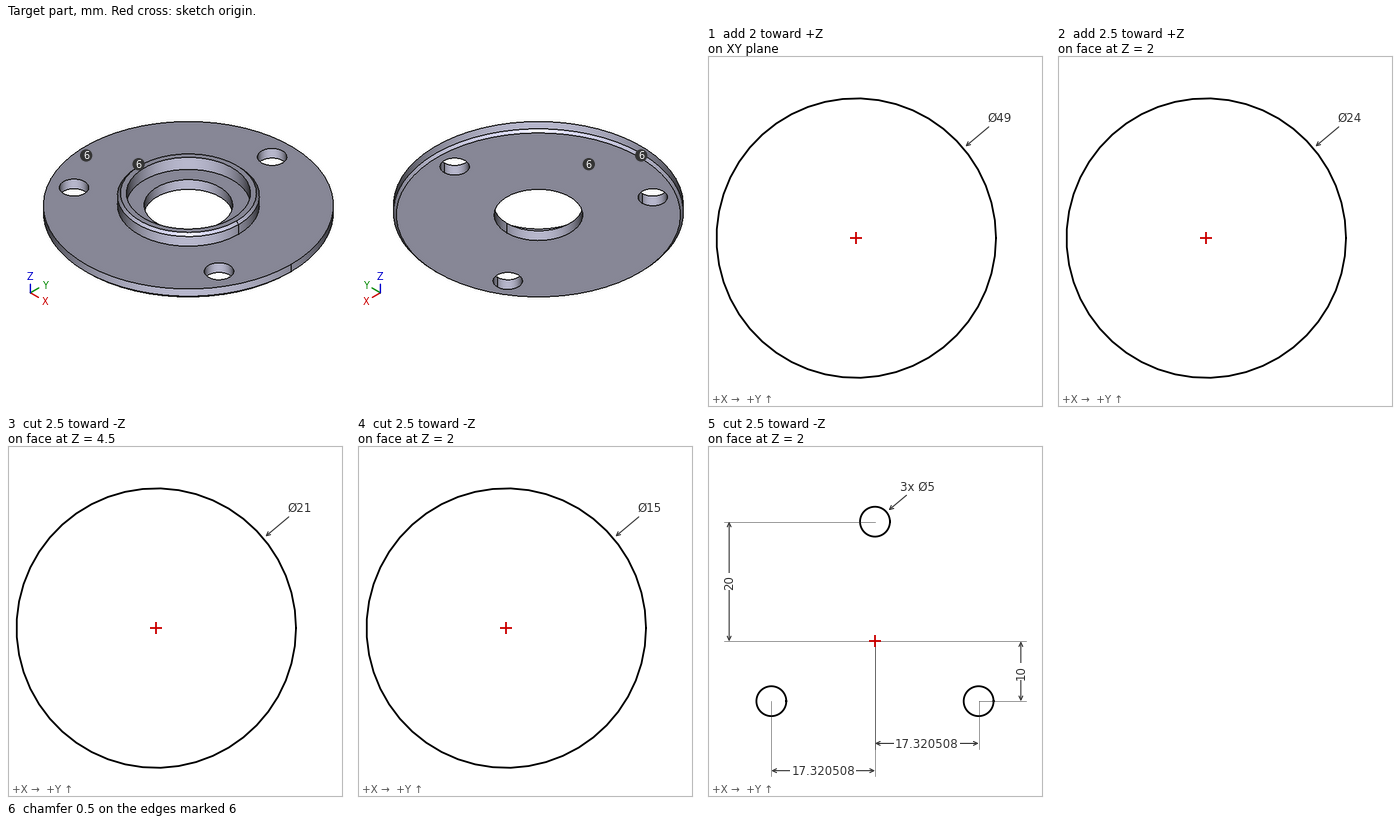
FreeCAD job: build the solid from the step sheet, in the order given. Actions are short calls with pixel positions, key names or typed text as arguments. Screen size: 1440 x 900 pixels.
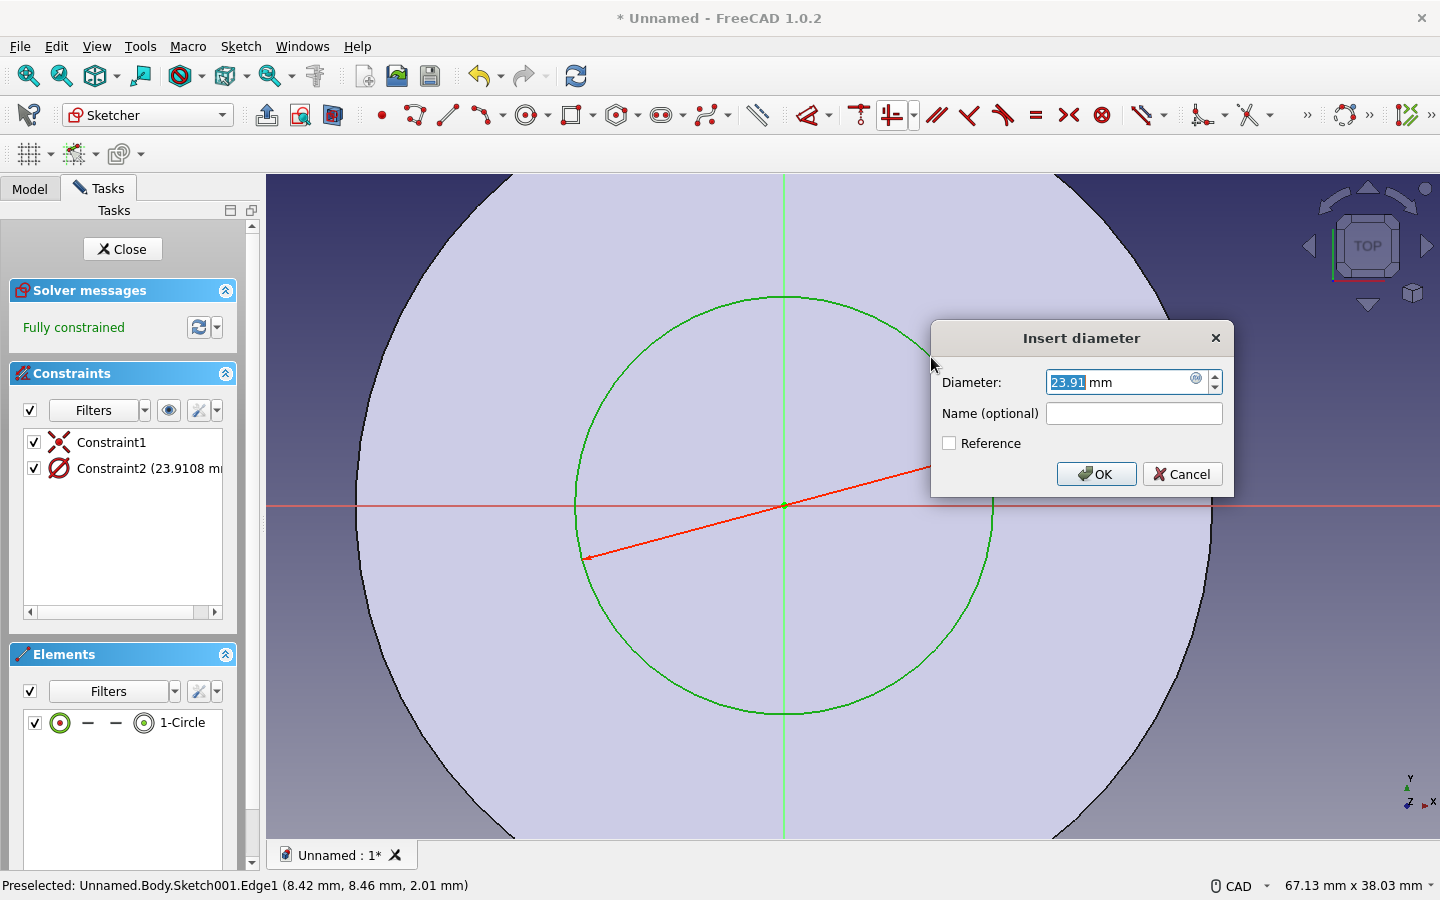
text(24)
key(Return)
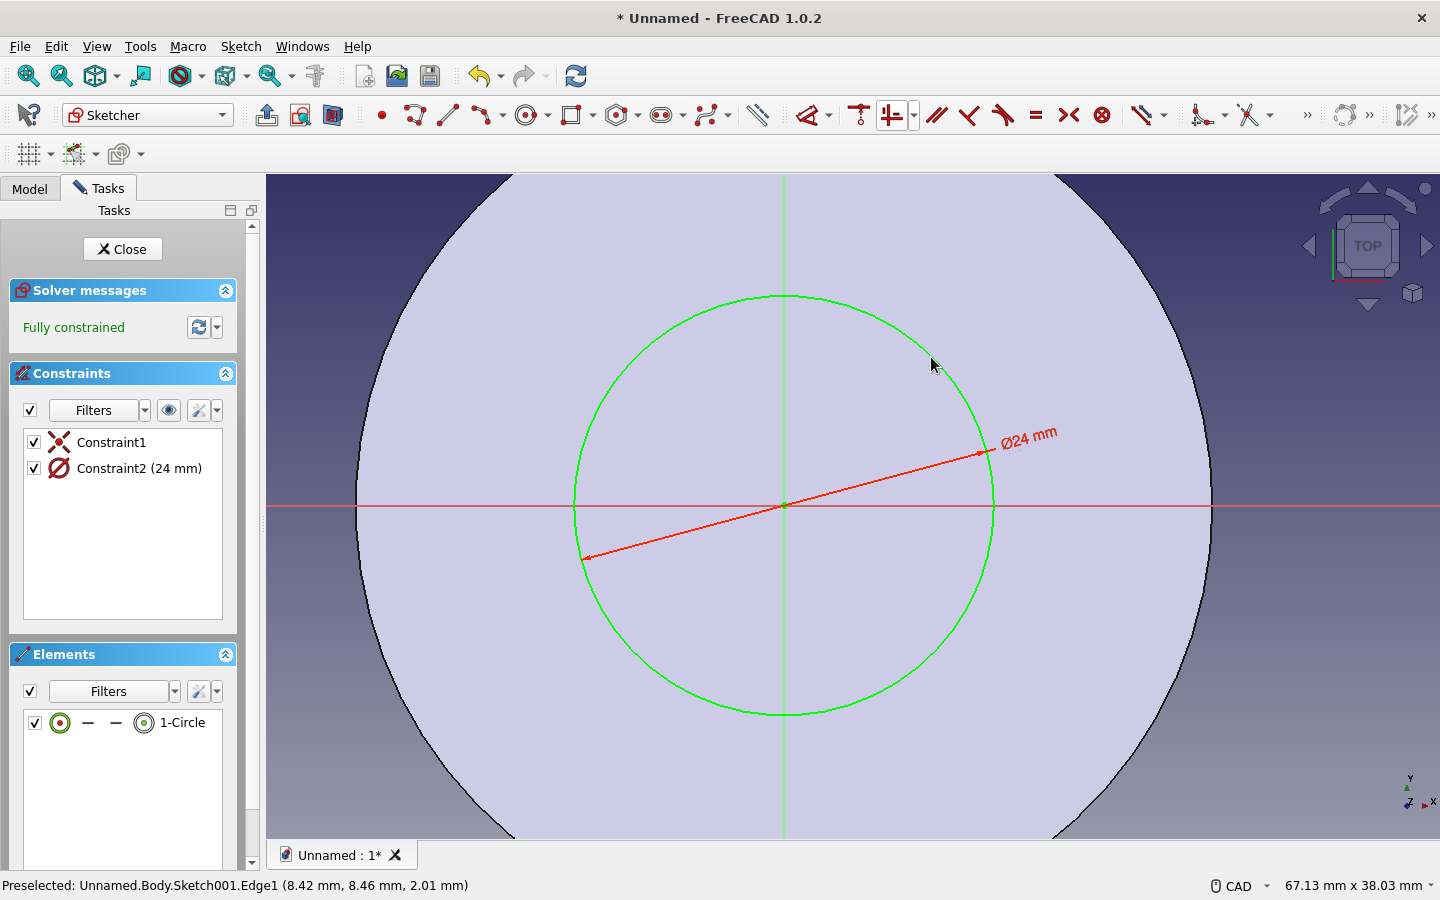
click(123, 249)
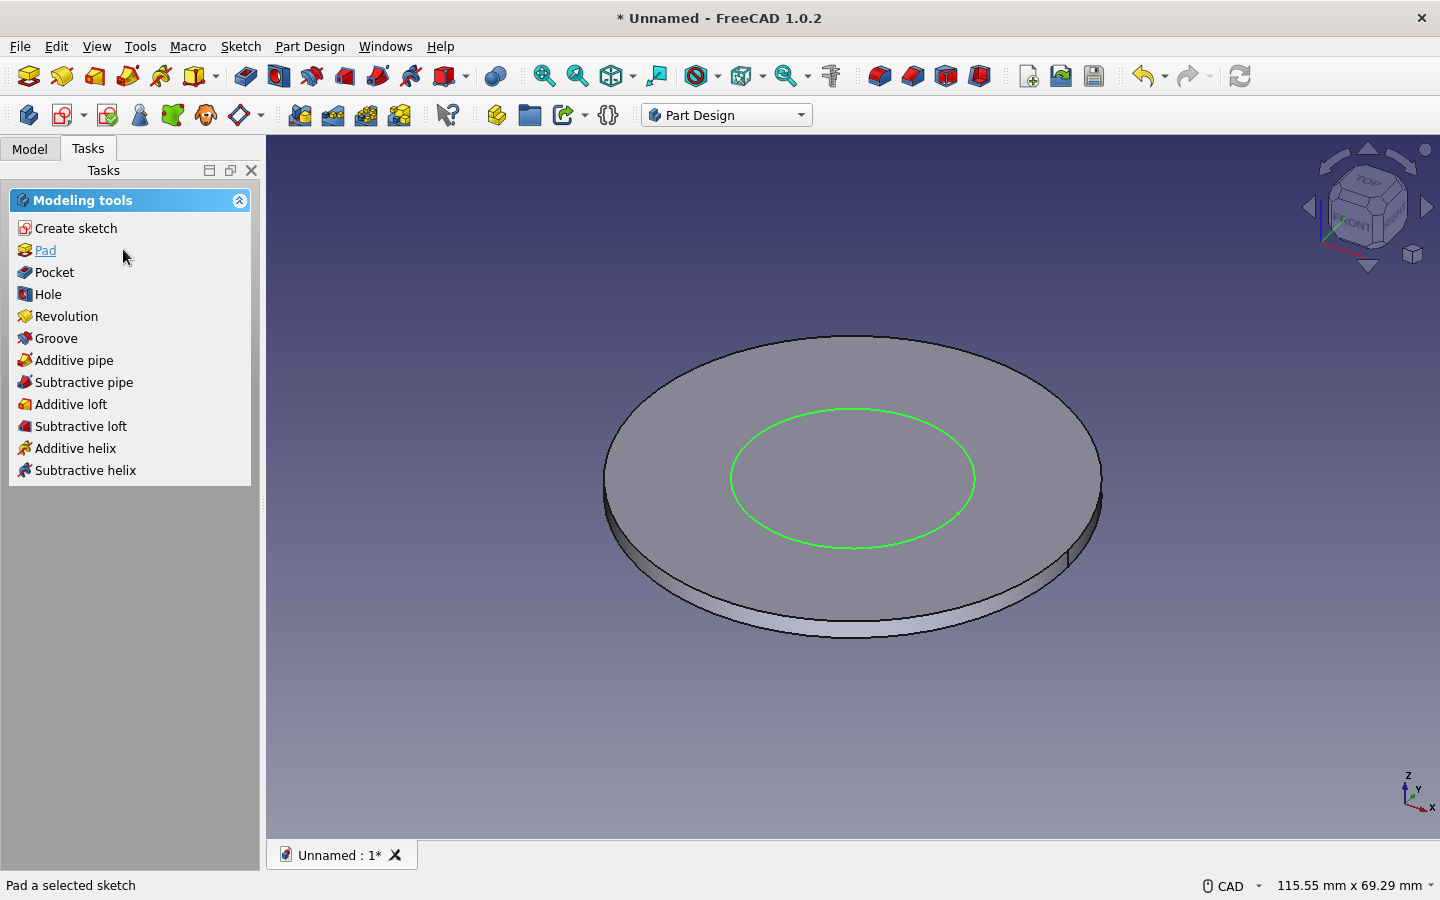
click(29, 76)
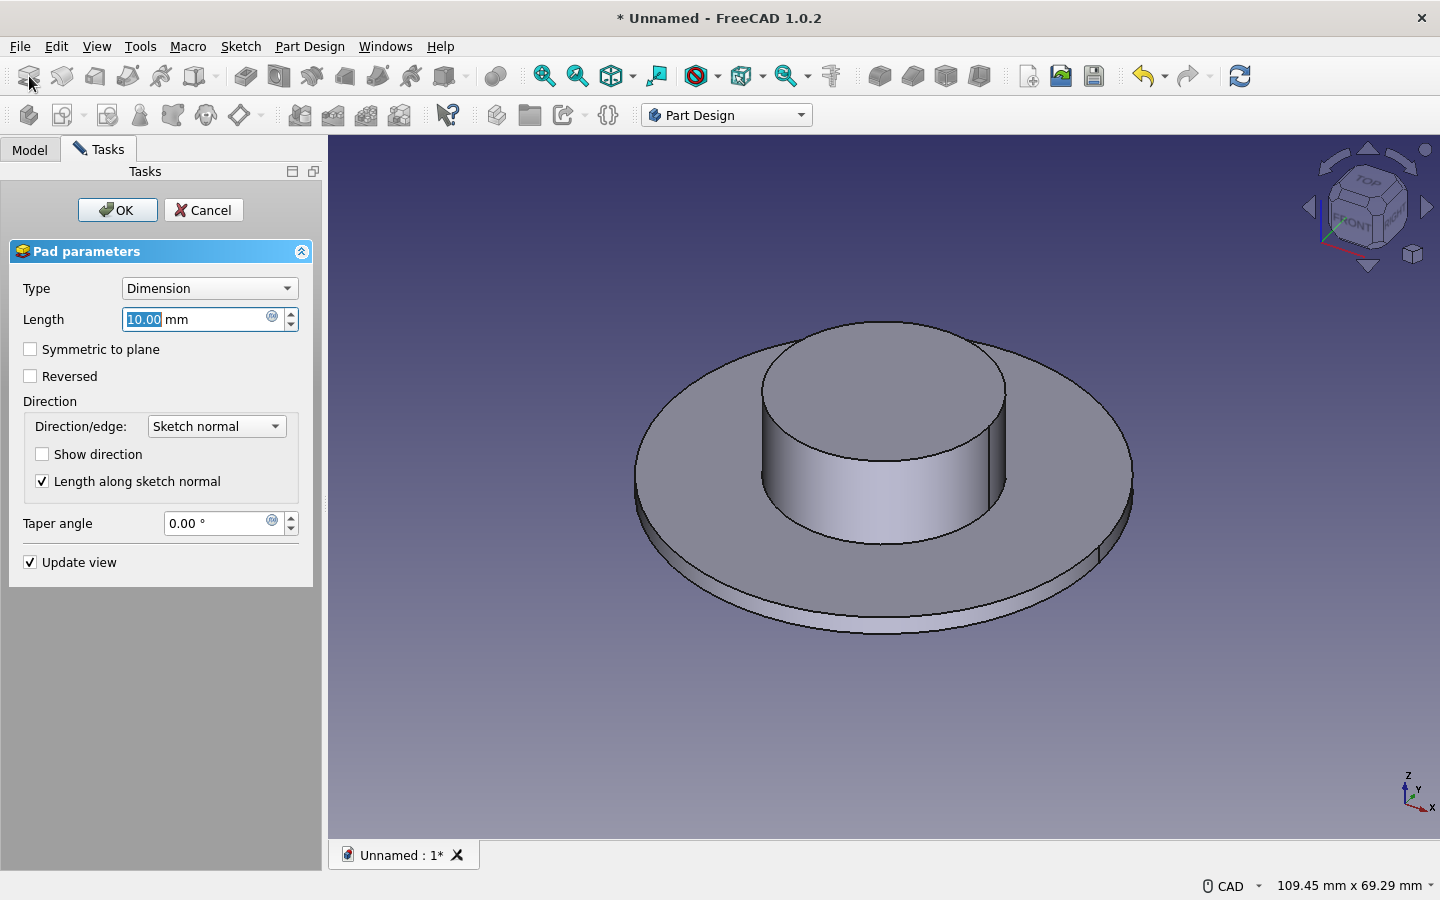
text(2.5)
key(Tab)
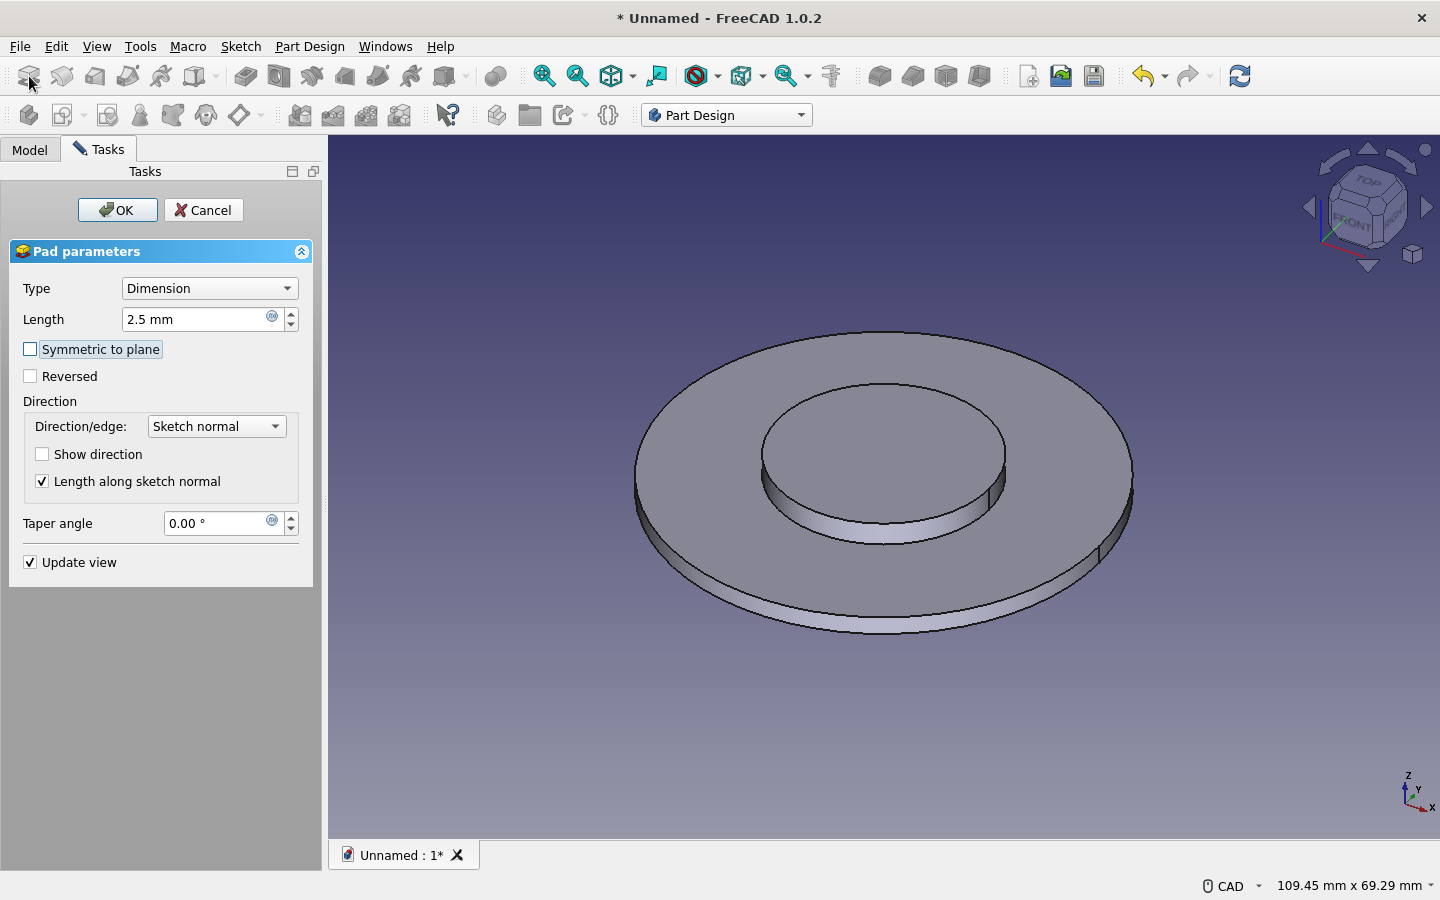
click(118, 210)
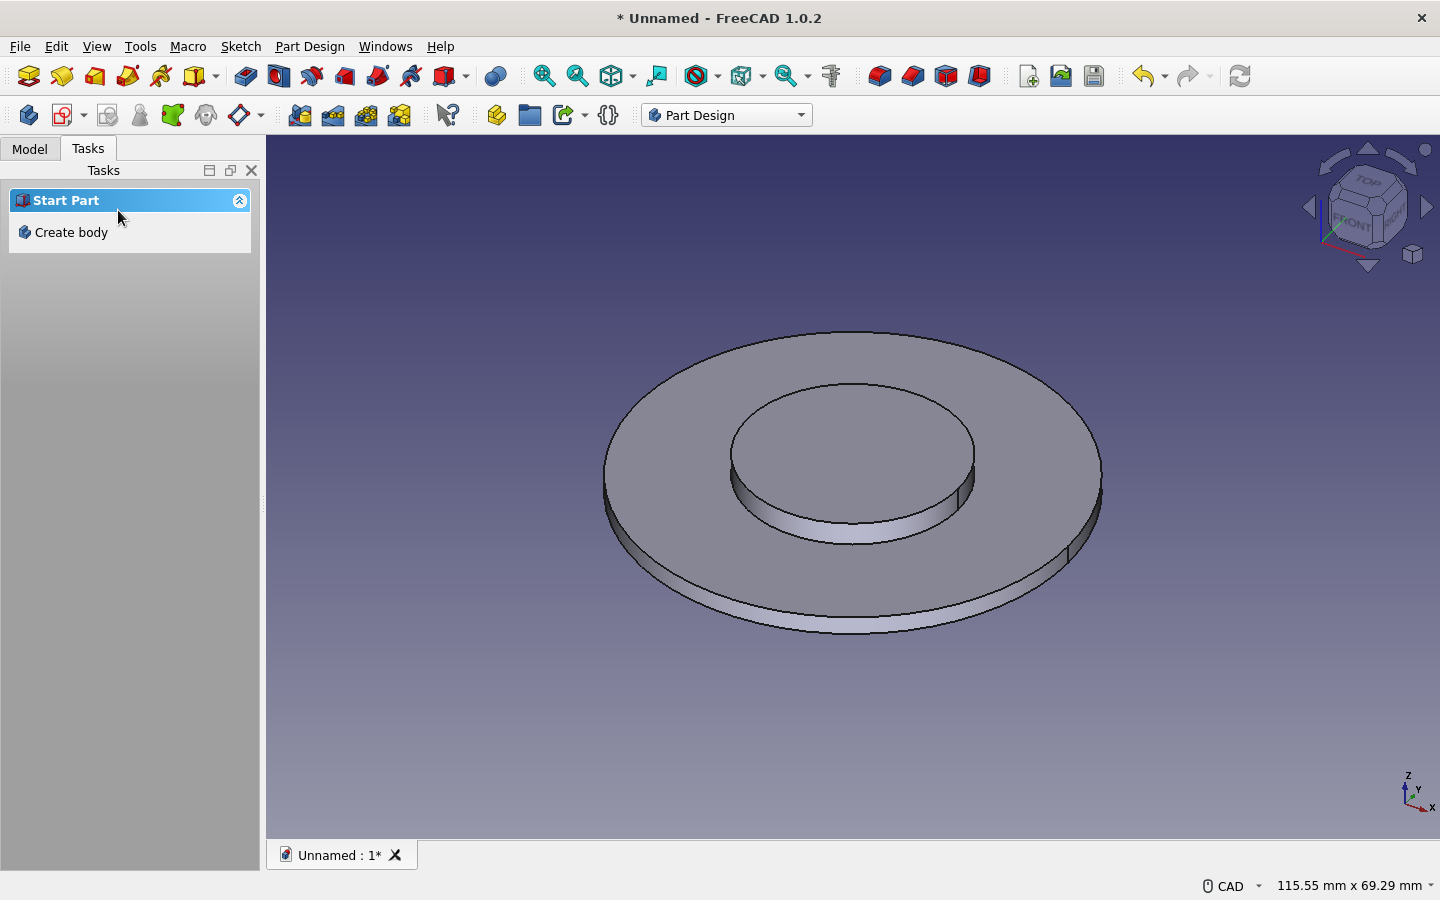
click(853, 453)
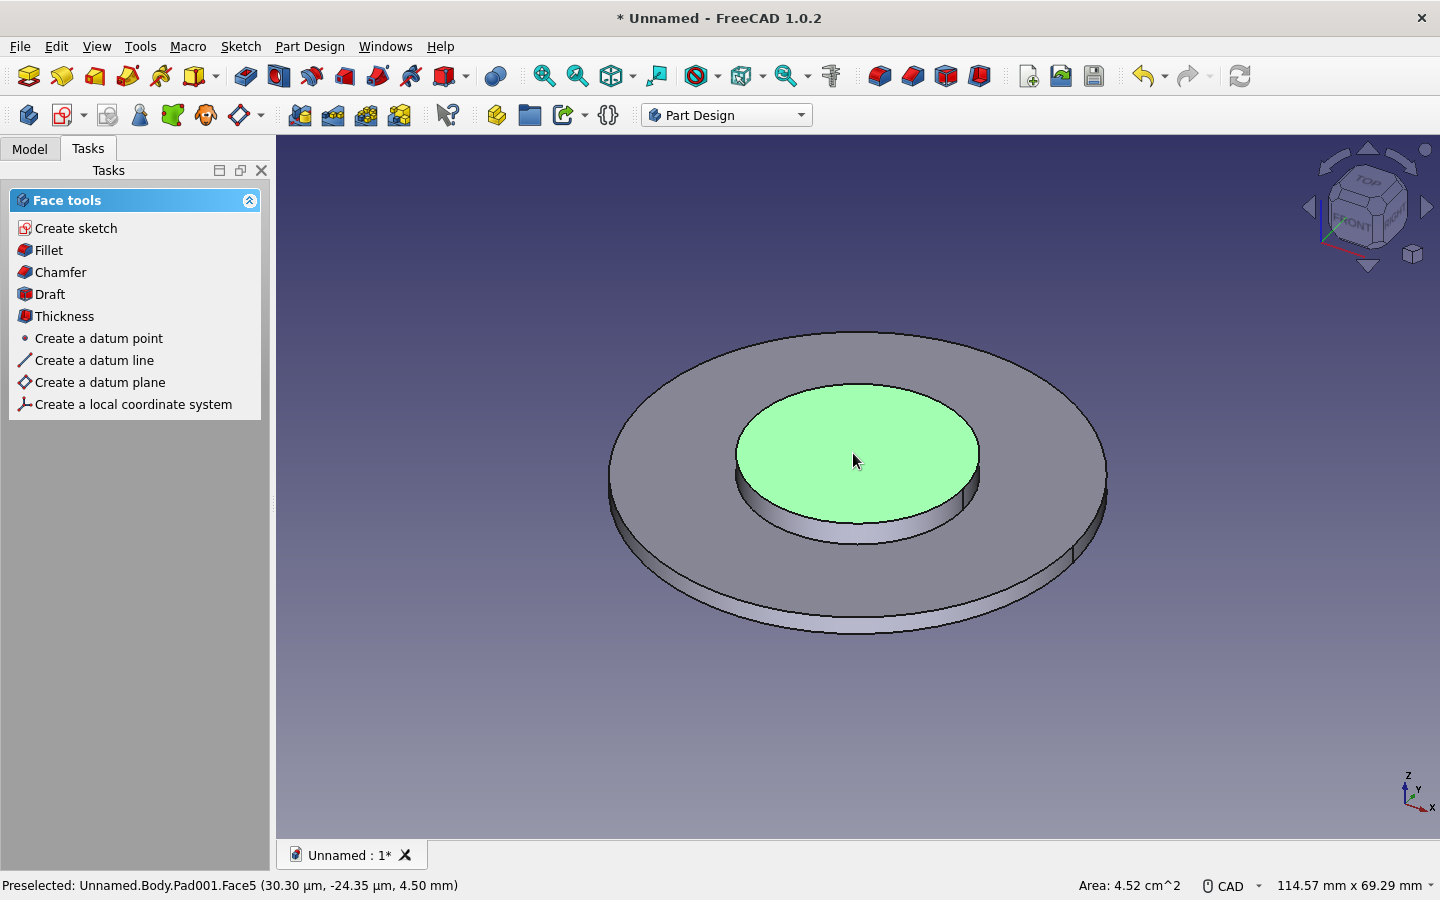
click(62, 116)